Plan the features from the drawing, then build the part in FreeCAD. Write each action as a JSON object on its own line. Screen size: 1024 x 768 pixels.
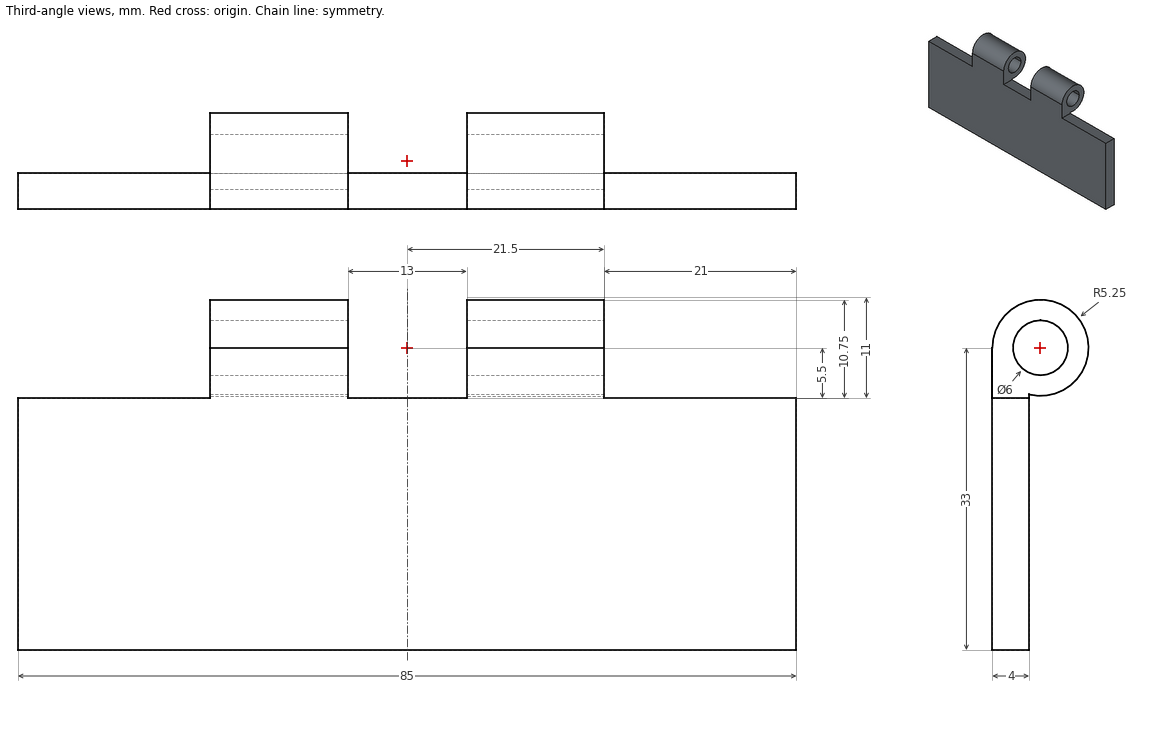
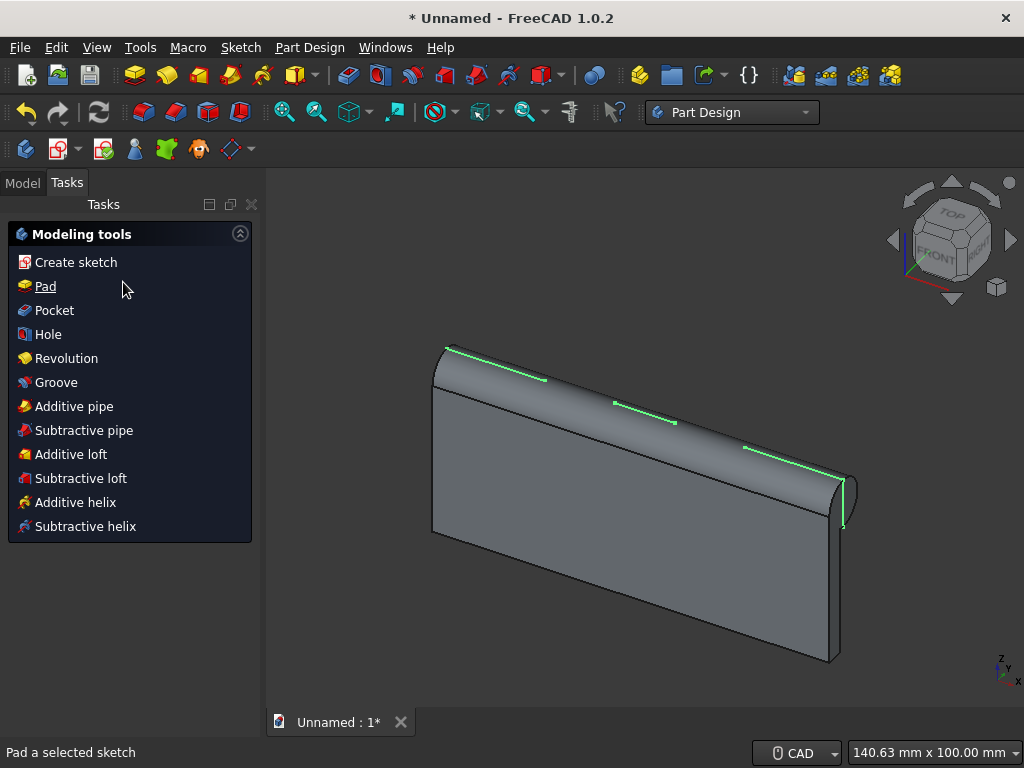
{"action": "left_click", "coordinate": [350, 76]}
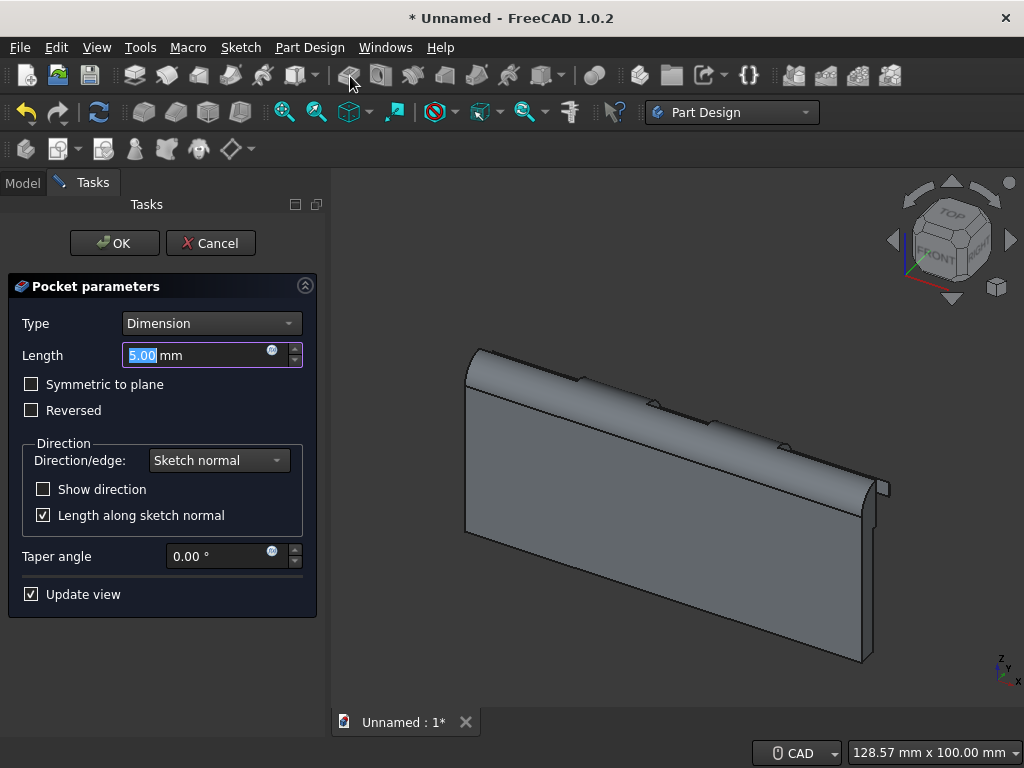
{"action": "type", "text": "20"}
{"action": "key", "text": "Tab"}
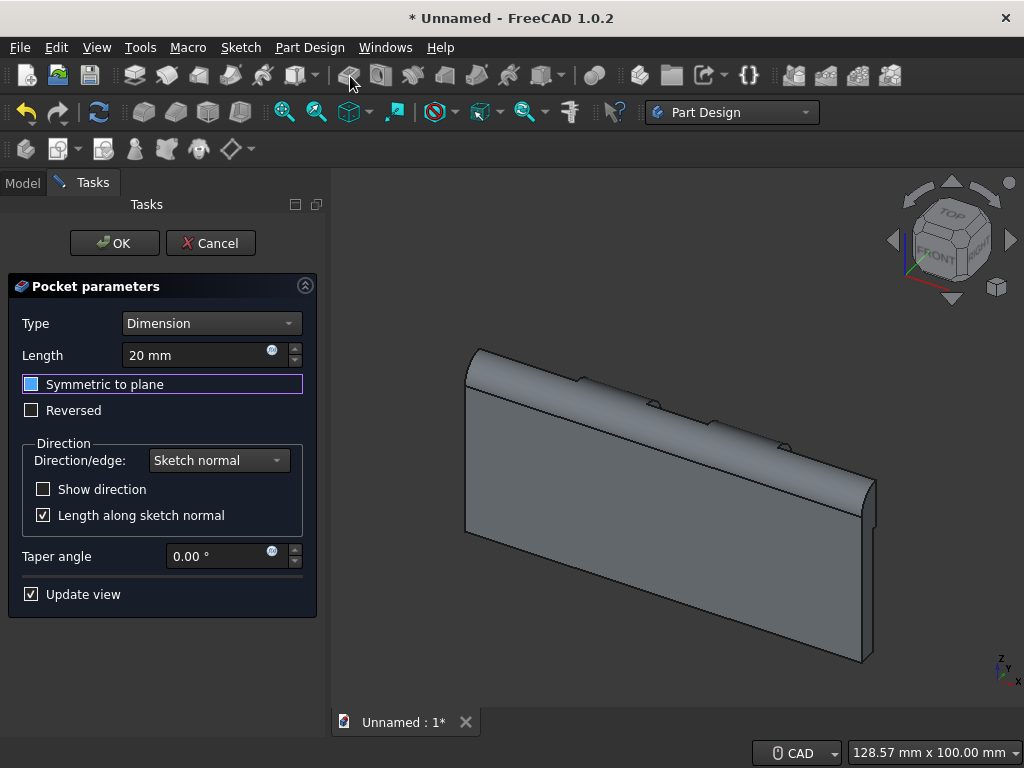
{"action": "left_click", "coordinate": [30, 384]}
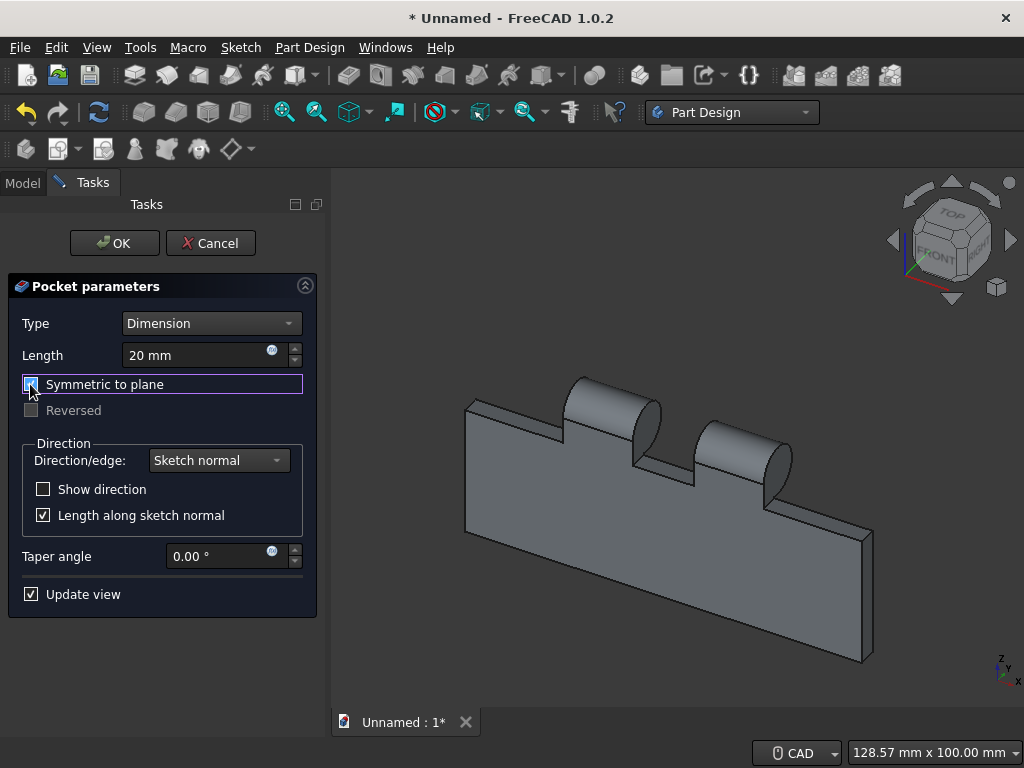
{"action": "left_click", "coordinate": [115, 243]}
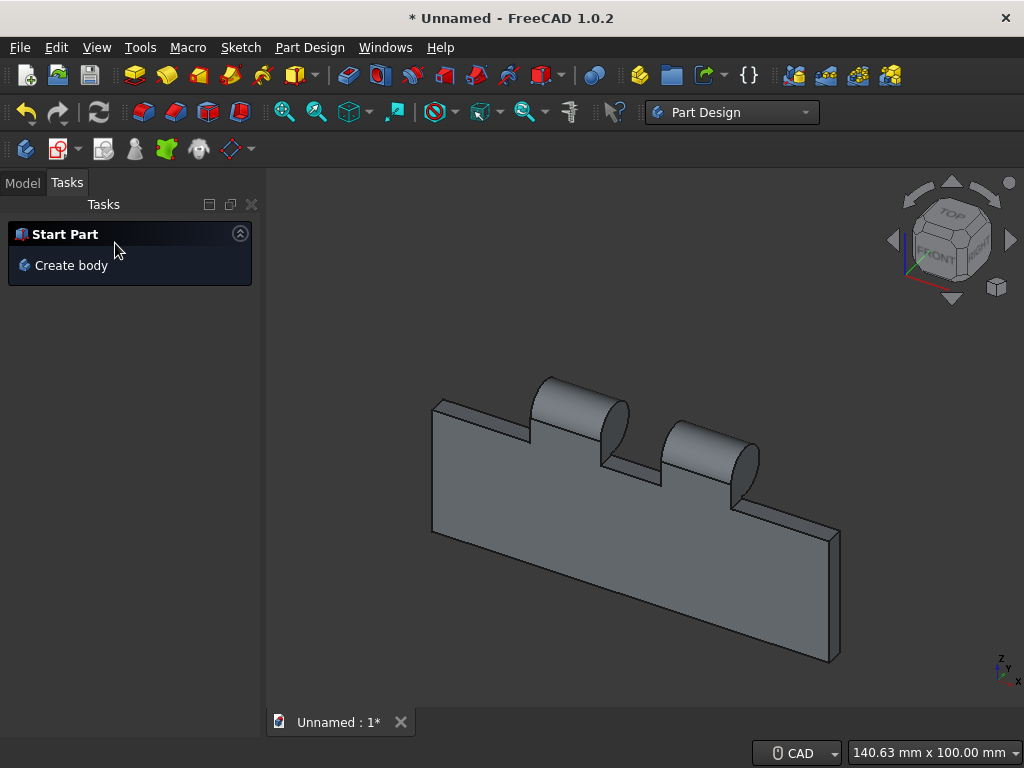
{"action": "key", "text": "6"}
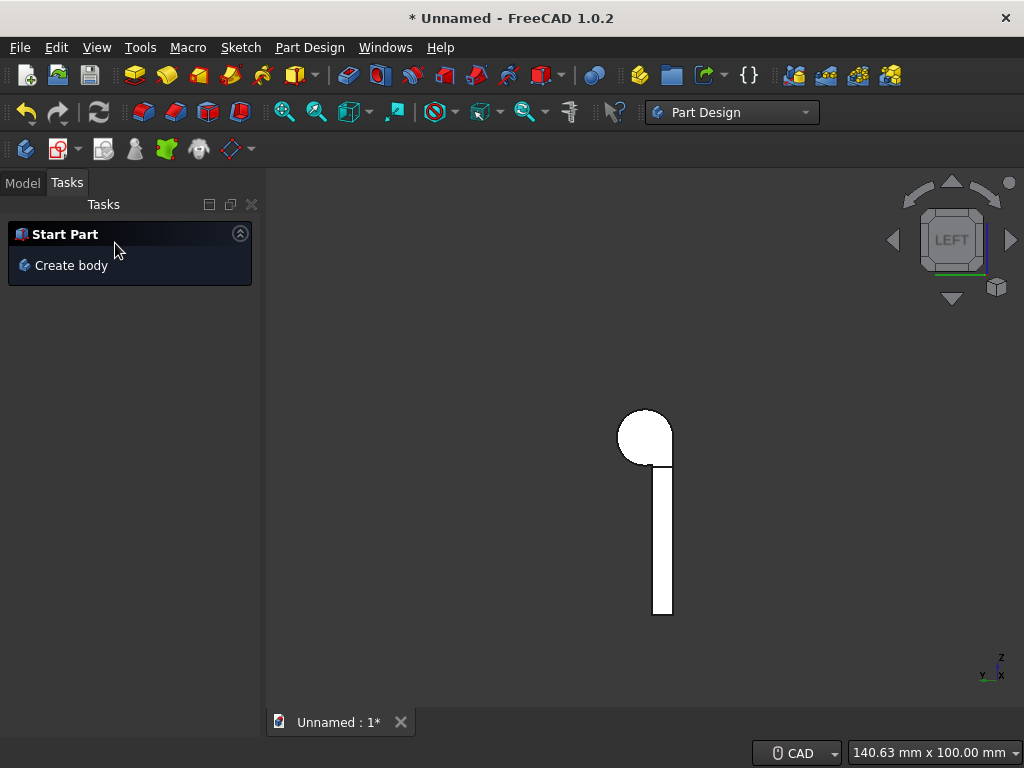
{"action": "left_click", "coordinate": [286, 112]}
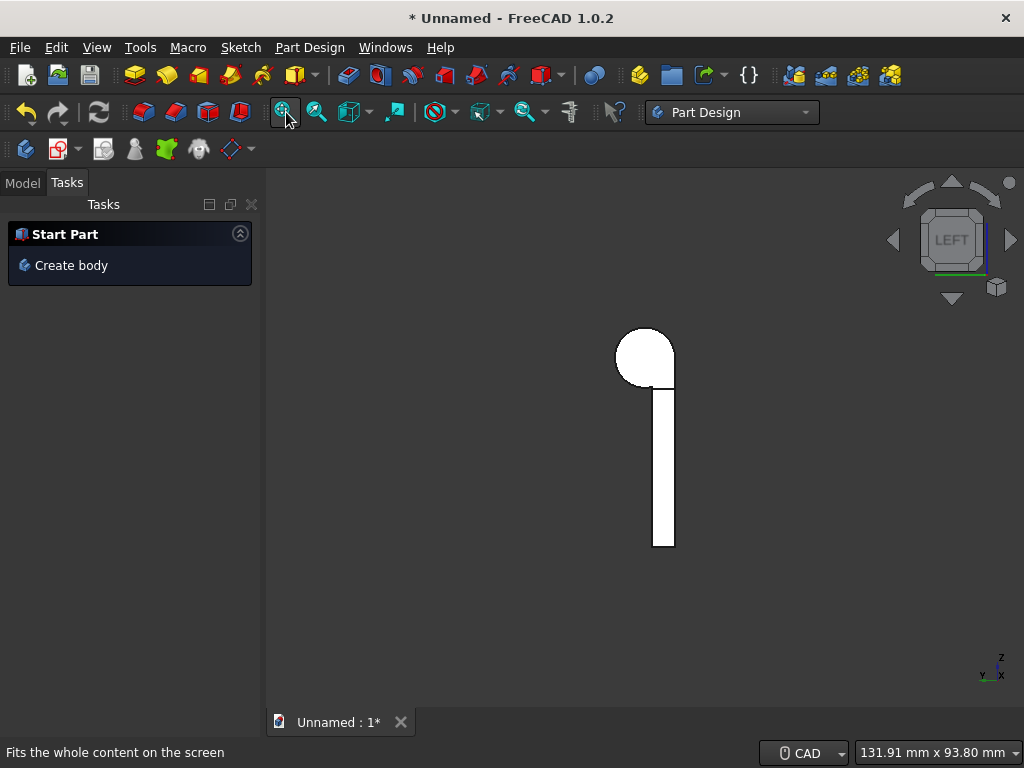
{"action": "left_click", "coordinate": [645, 357]}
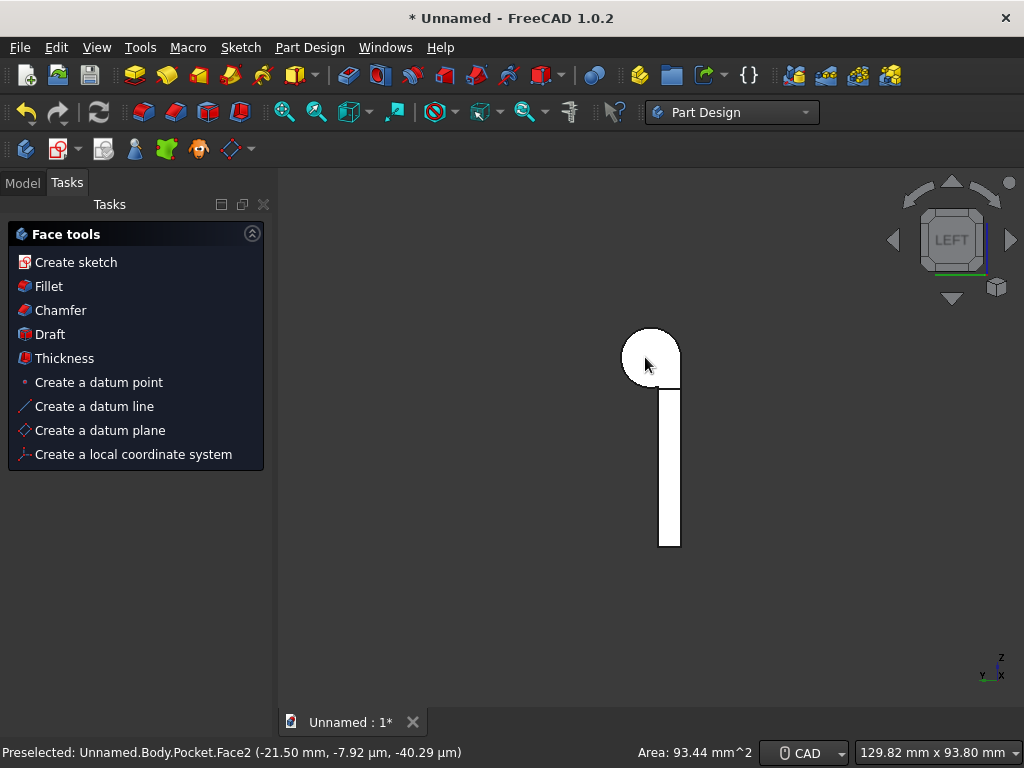
{"action": "left_click", "coordinate": [58, 150]}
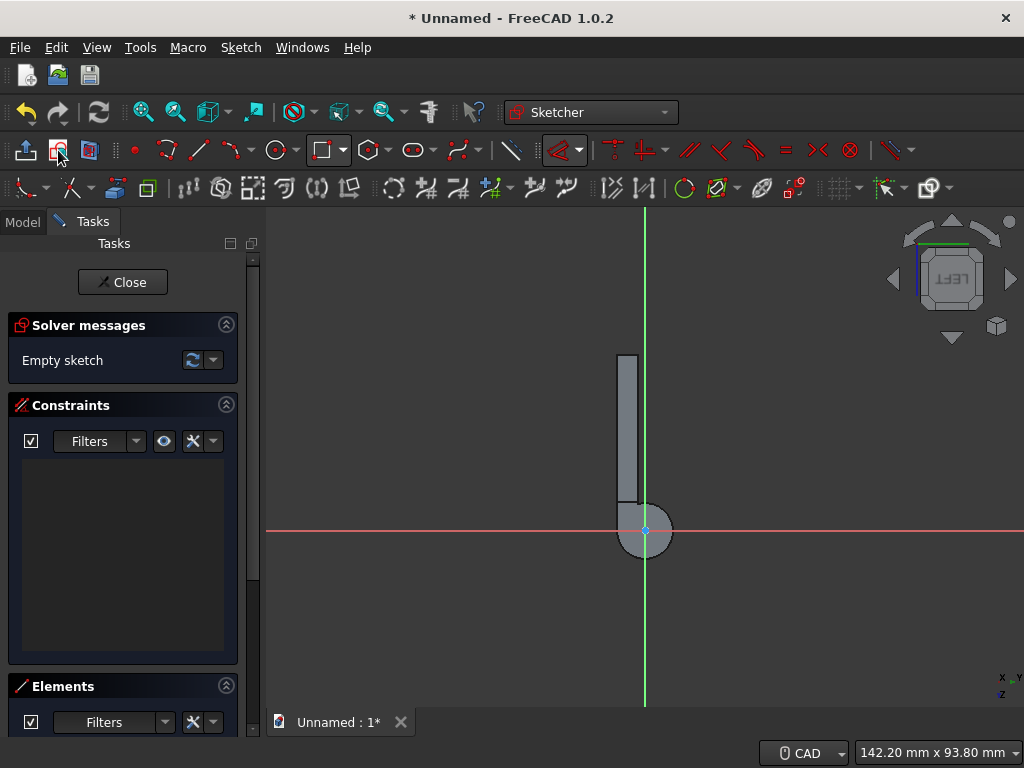
{"action": "scroll", "coordinate": [654, 540], "scroll_direction": "up", "scroll_amount": 11}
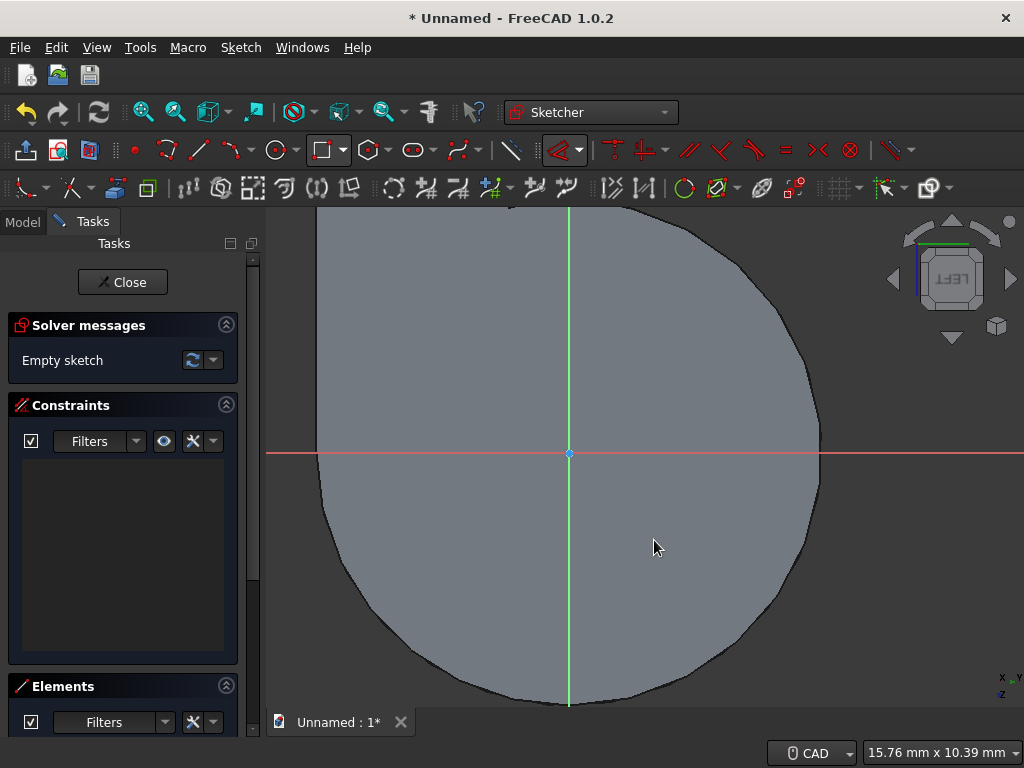
{"action": "left_click", "coordinate": [276, 150]}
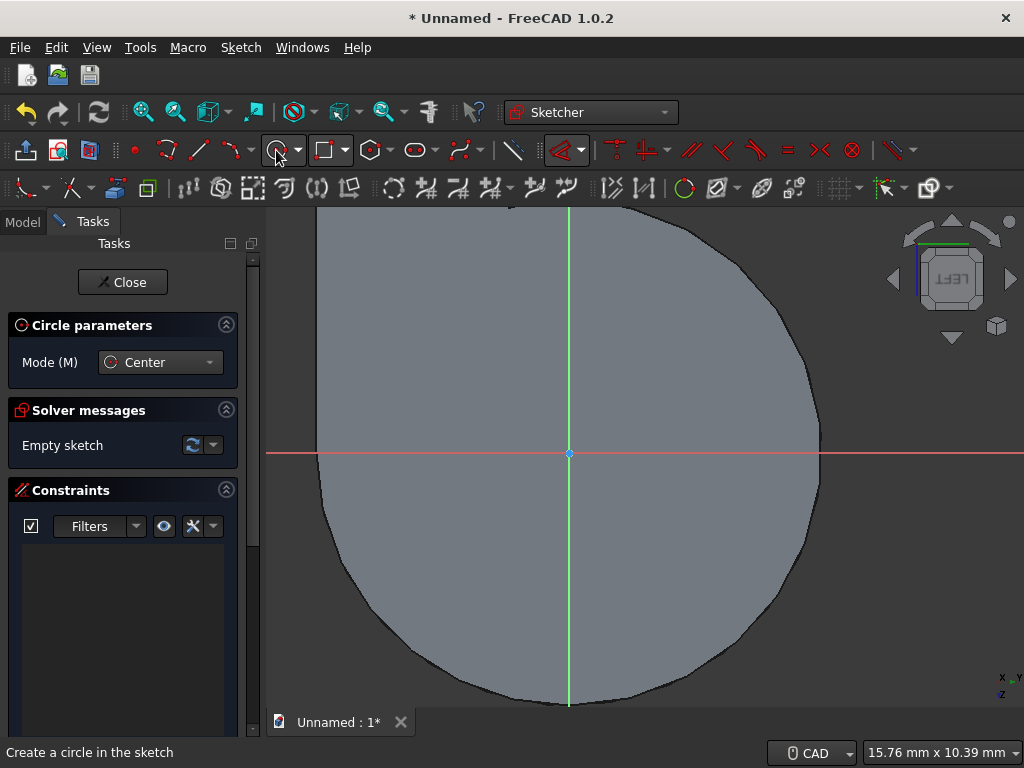
{"action": "left_click", "coordinate": [569, 453]}
{"action": "left_click", "coordinate": [671, 351]}
{"action": "key", "text": "Escape"}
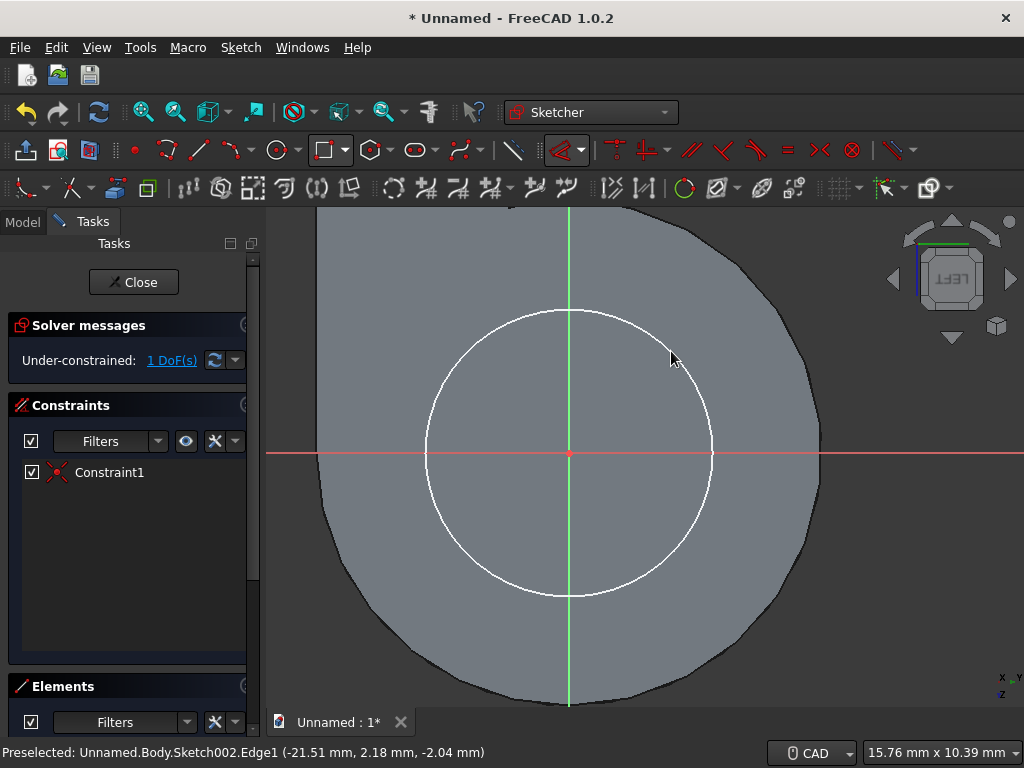
{"action": "left_click", "coordinate": [670, 351]}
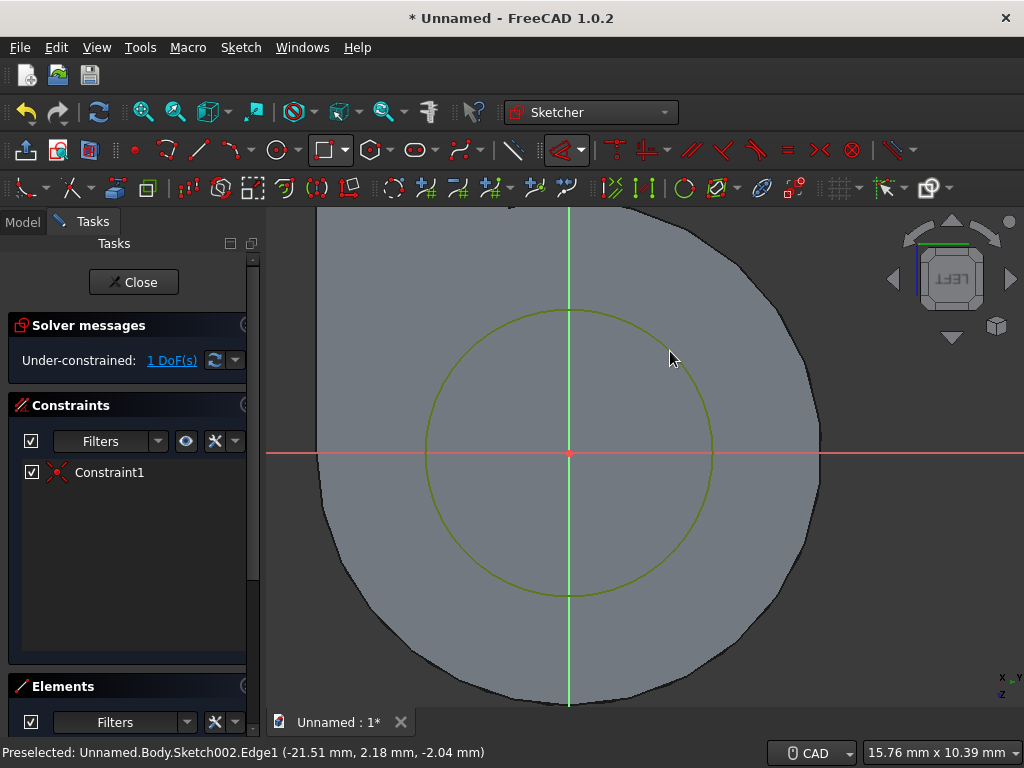
{"action": "left_click", "coordinate": [584, 150]}